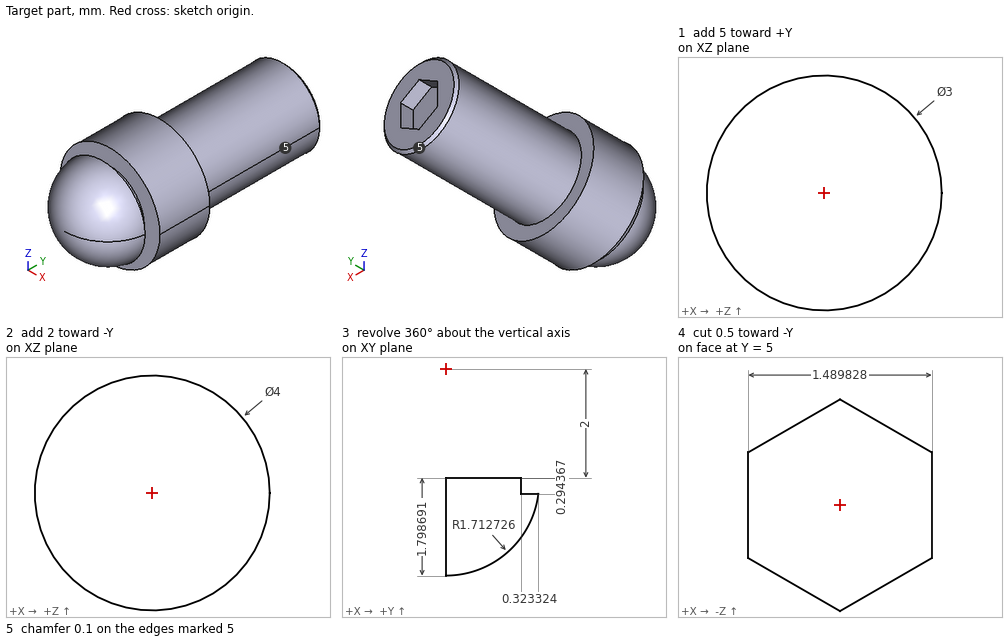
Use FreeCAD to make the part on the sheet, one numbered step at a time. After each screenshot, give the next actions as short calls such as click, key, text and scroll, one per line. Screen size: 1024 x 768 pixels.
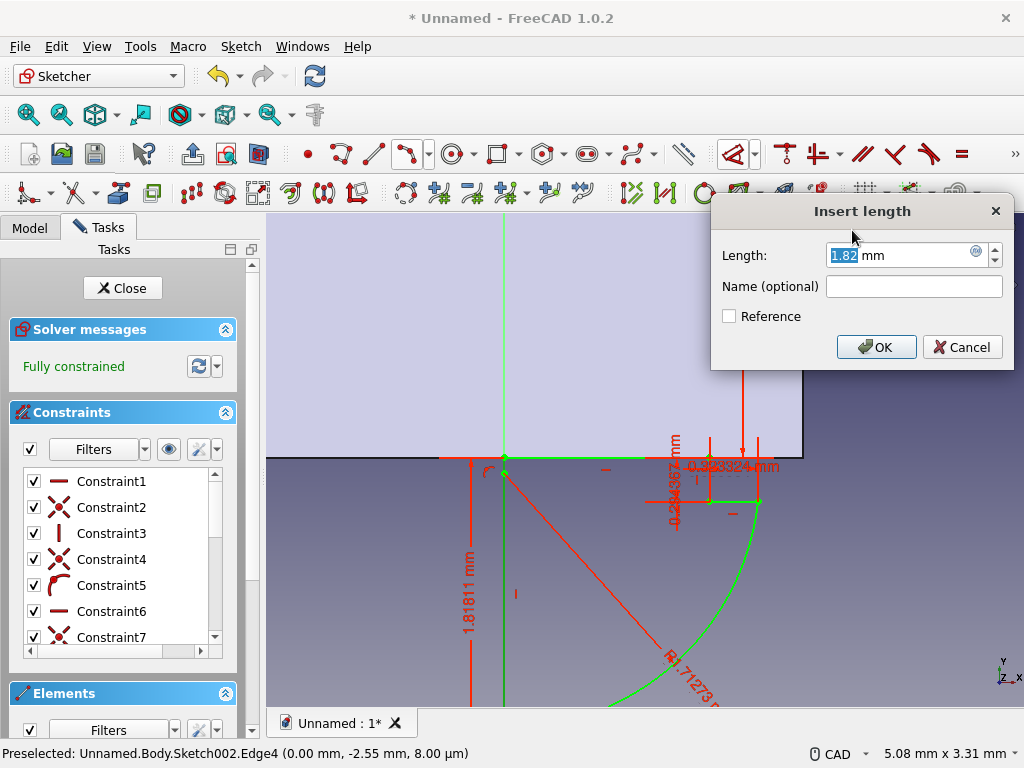
text(1.798691)
key(Return)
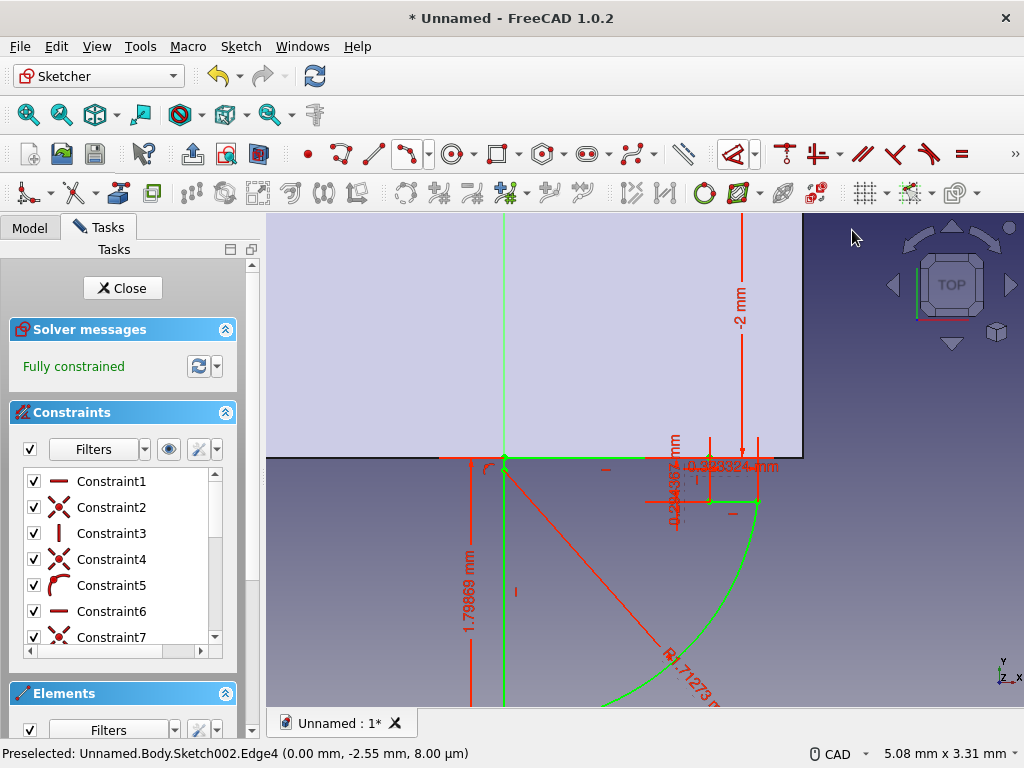
click(123, 288)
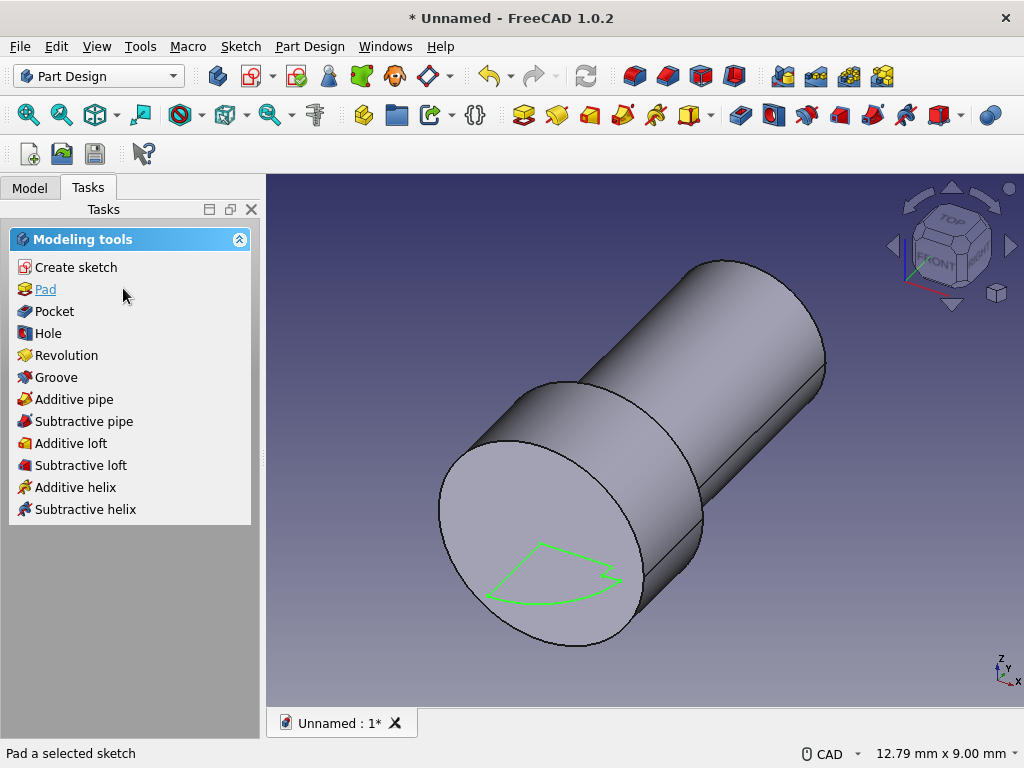
click(557, 116)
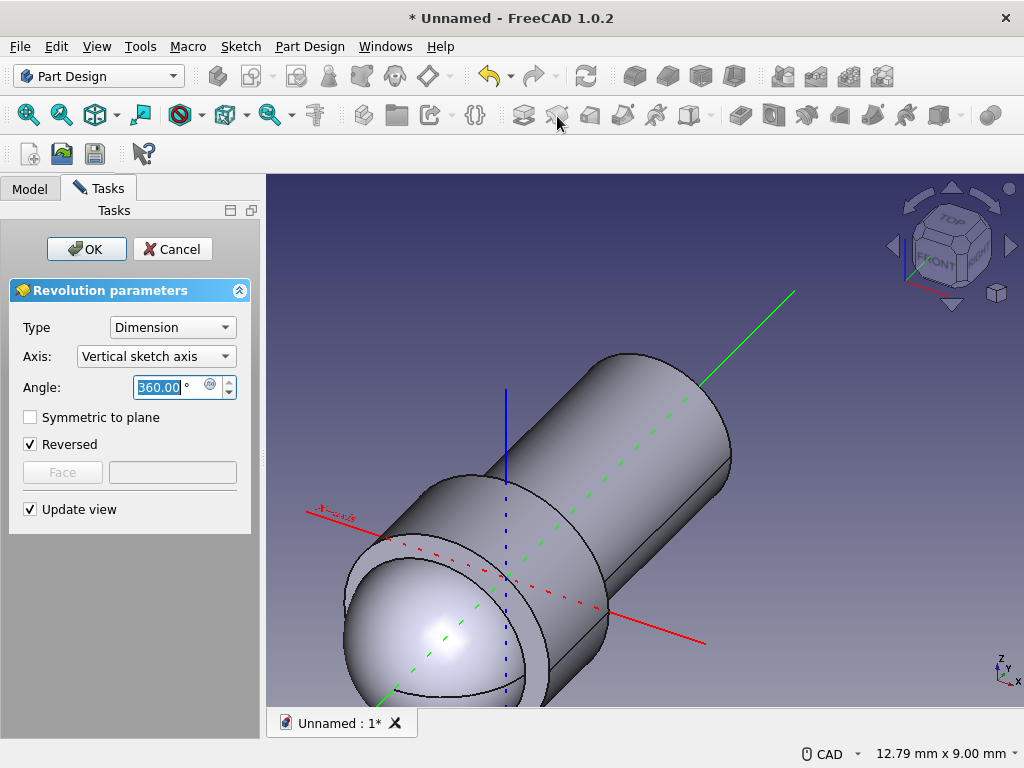
click(87, 249)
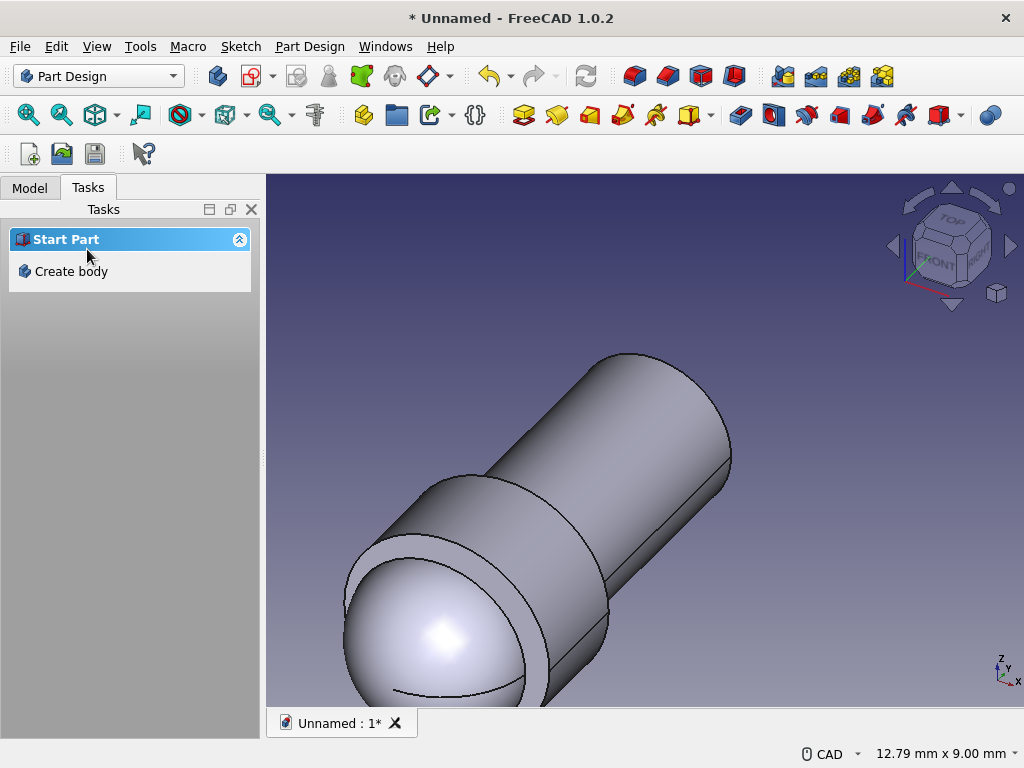
click(29, 116)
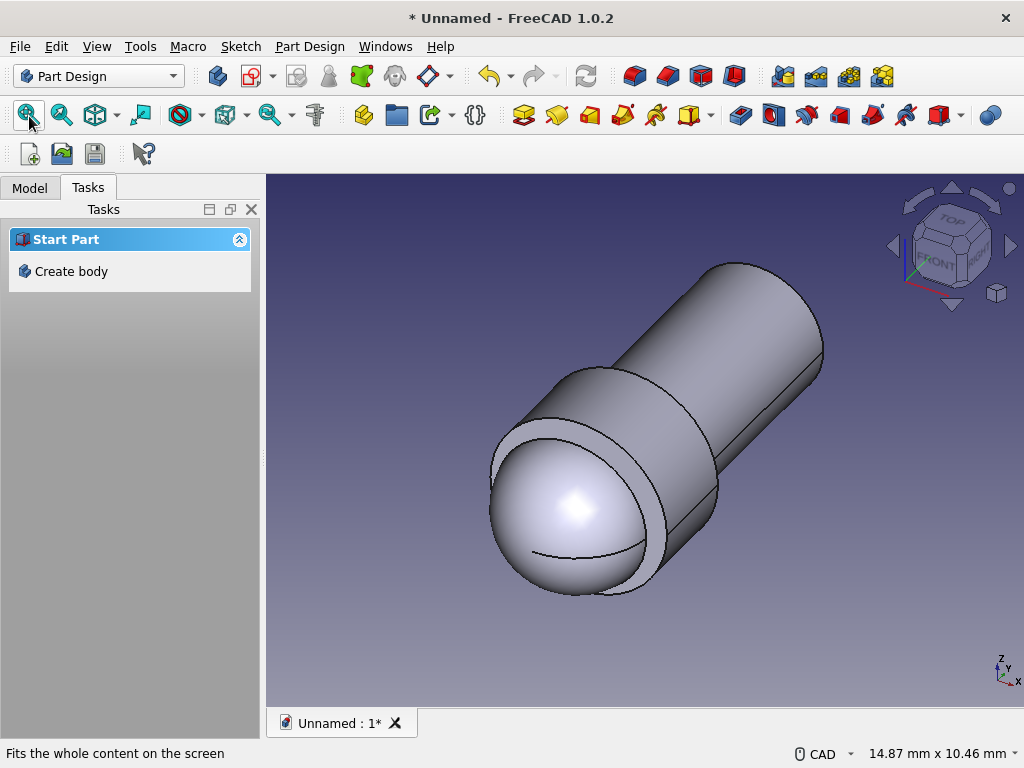
key(4)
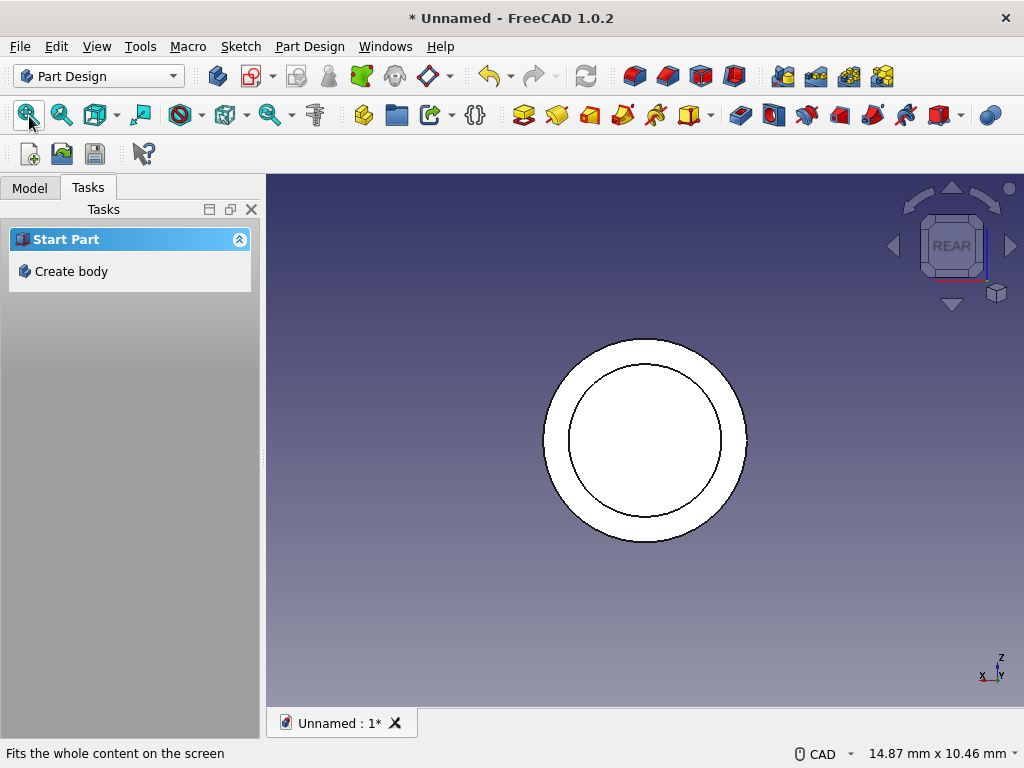
click(29, 116)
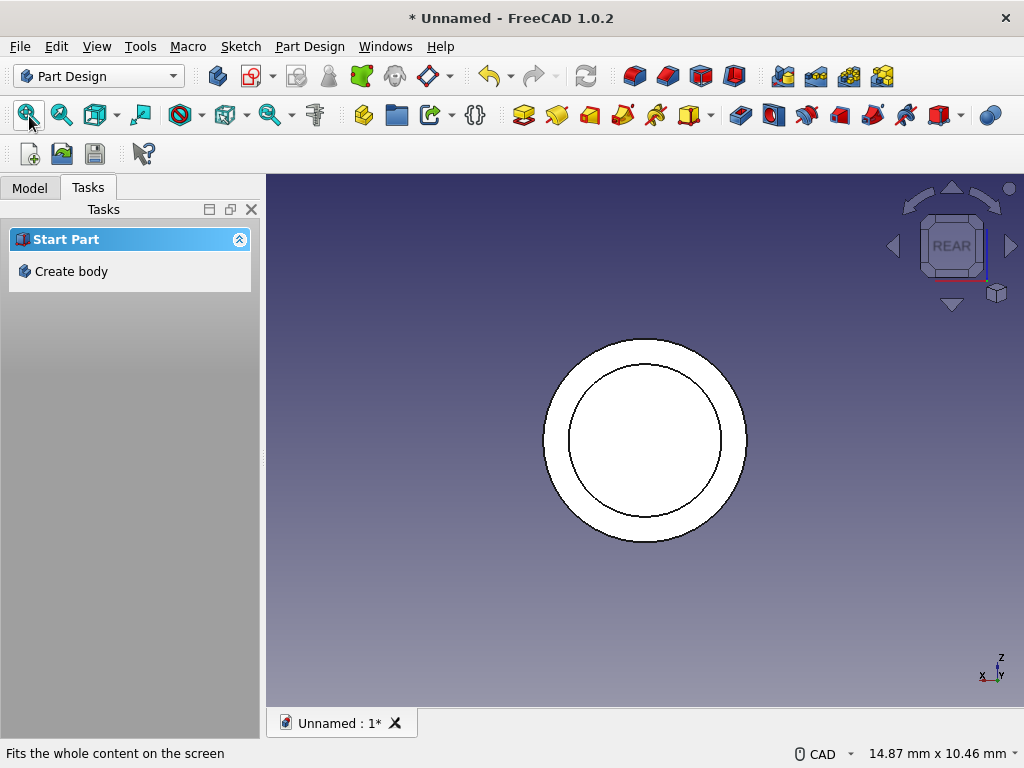
click(645, 440)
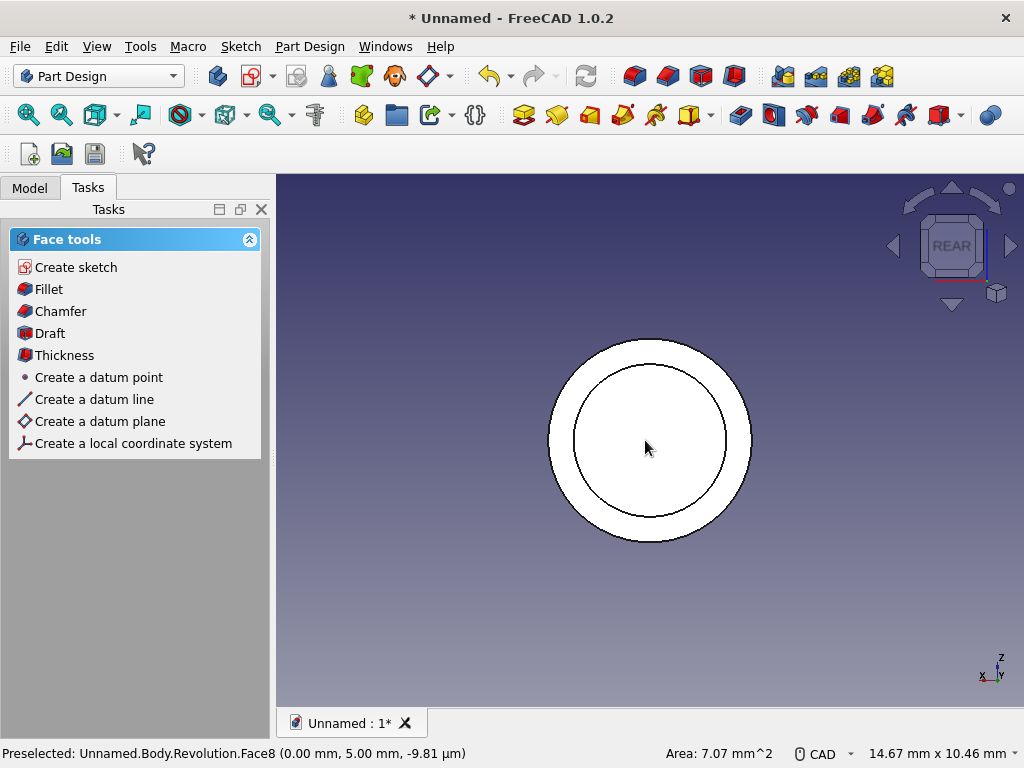
click(250, 76)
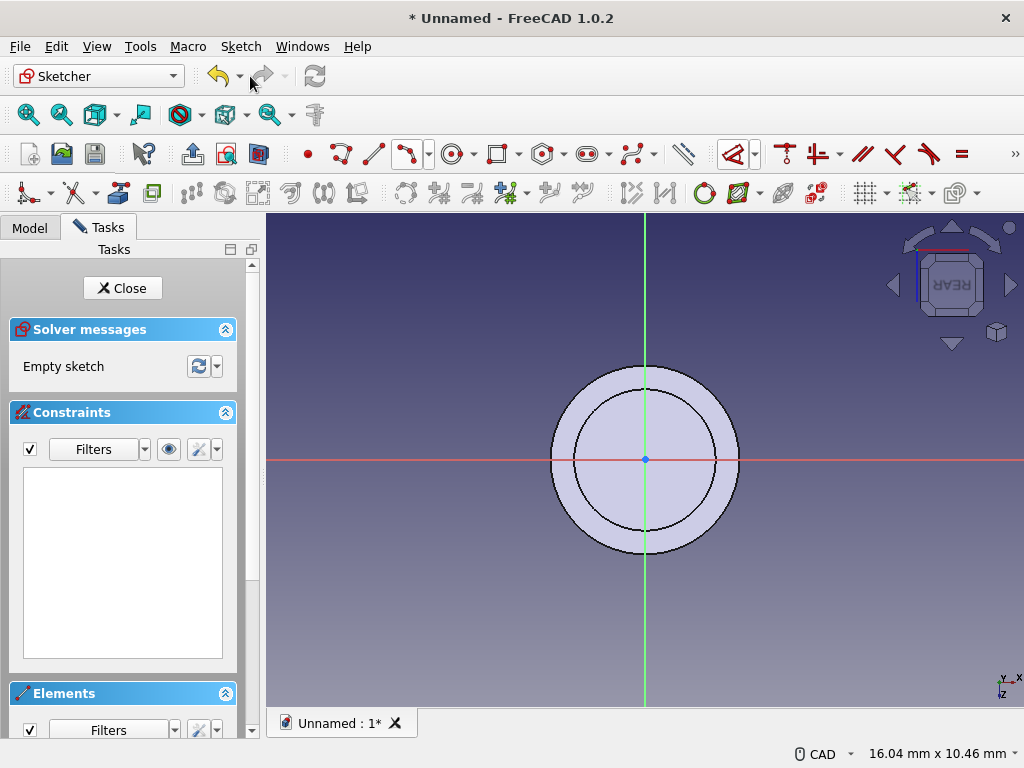
scroll(667, 460, up, 7)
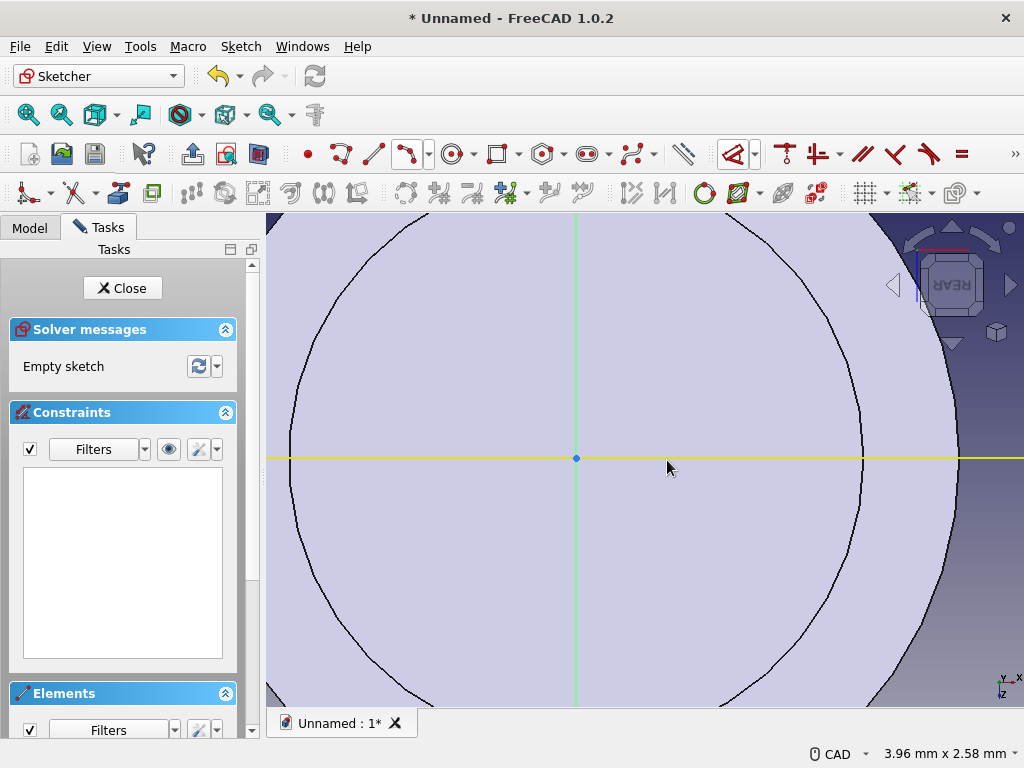
click(542, 154)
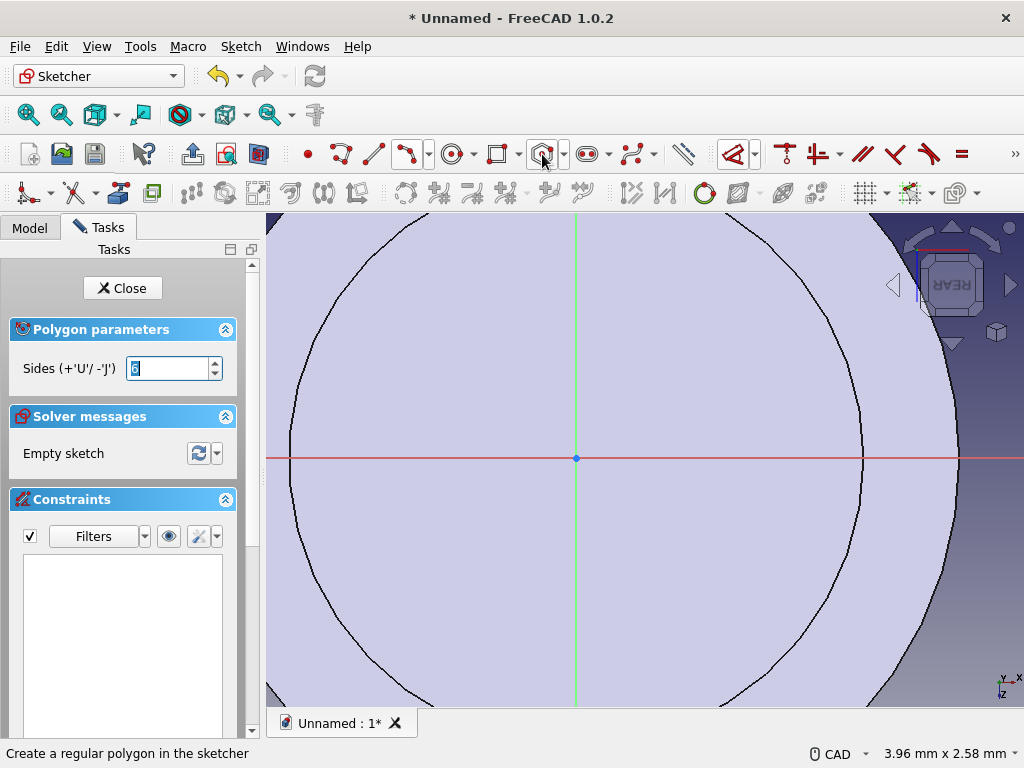
click(576, 458)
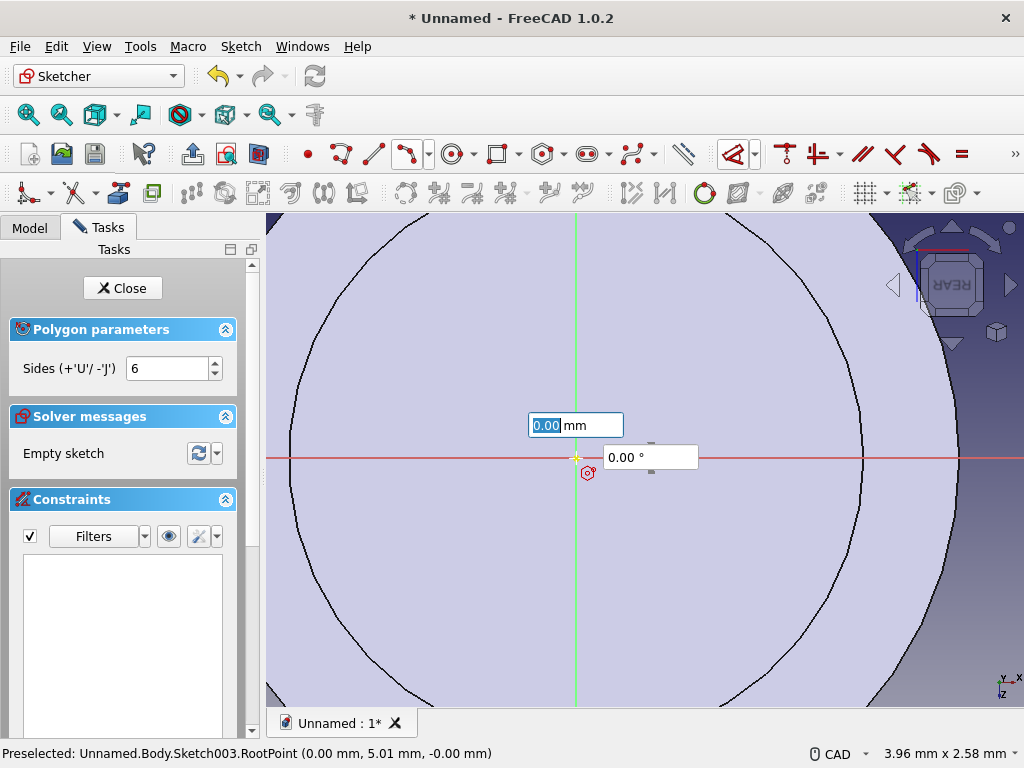
click(576, 294)
key(Escape)